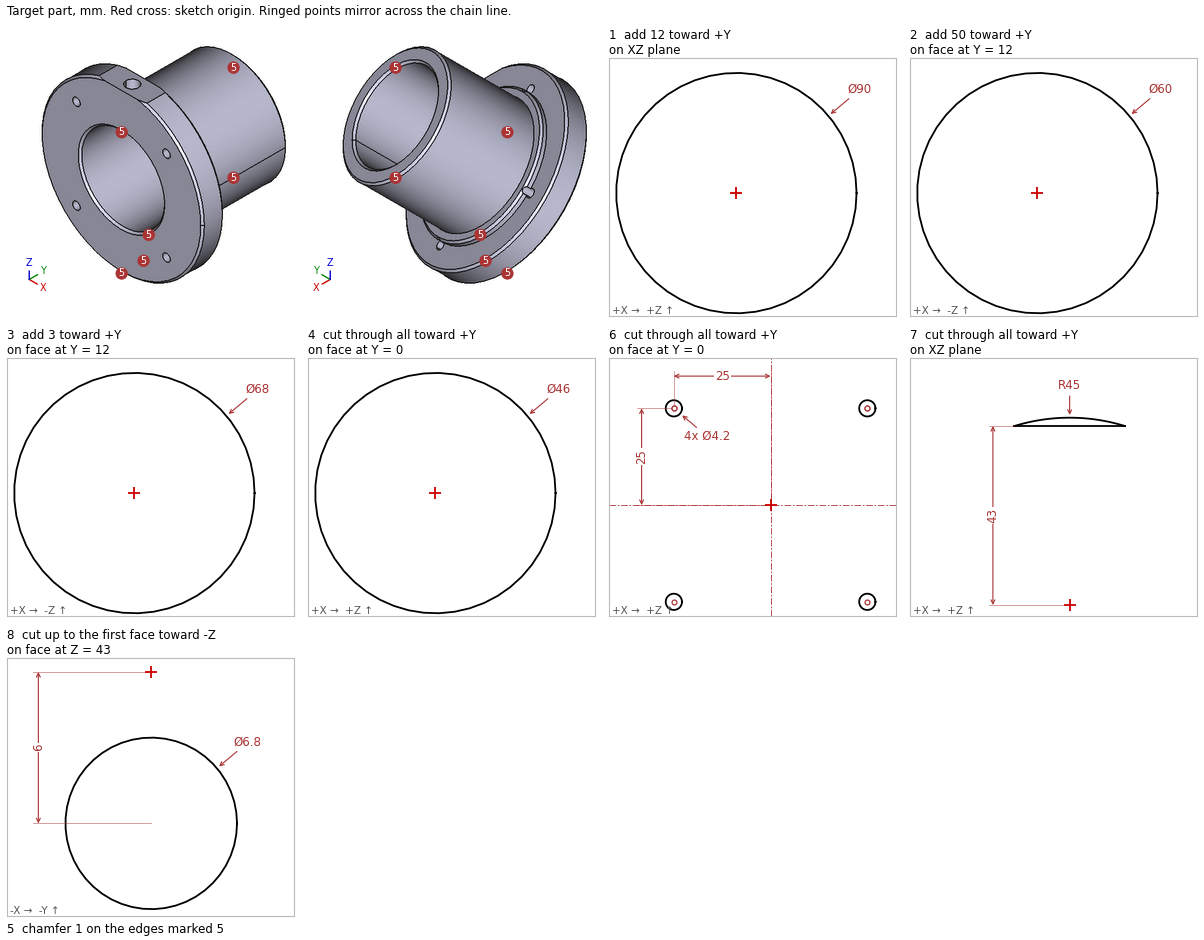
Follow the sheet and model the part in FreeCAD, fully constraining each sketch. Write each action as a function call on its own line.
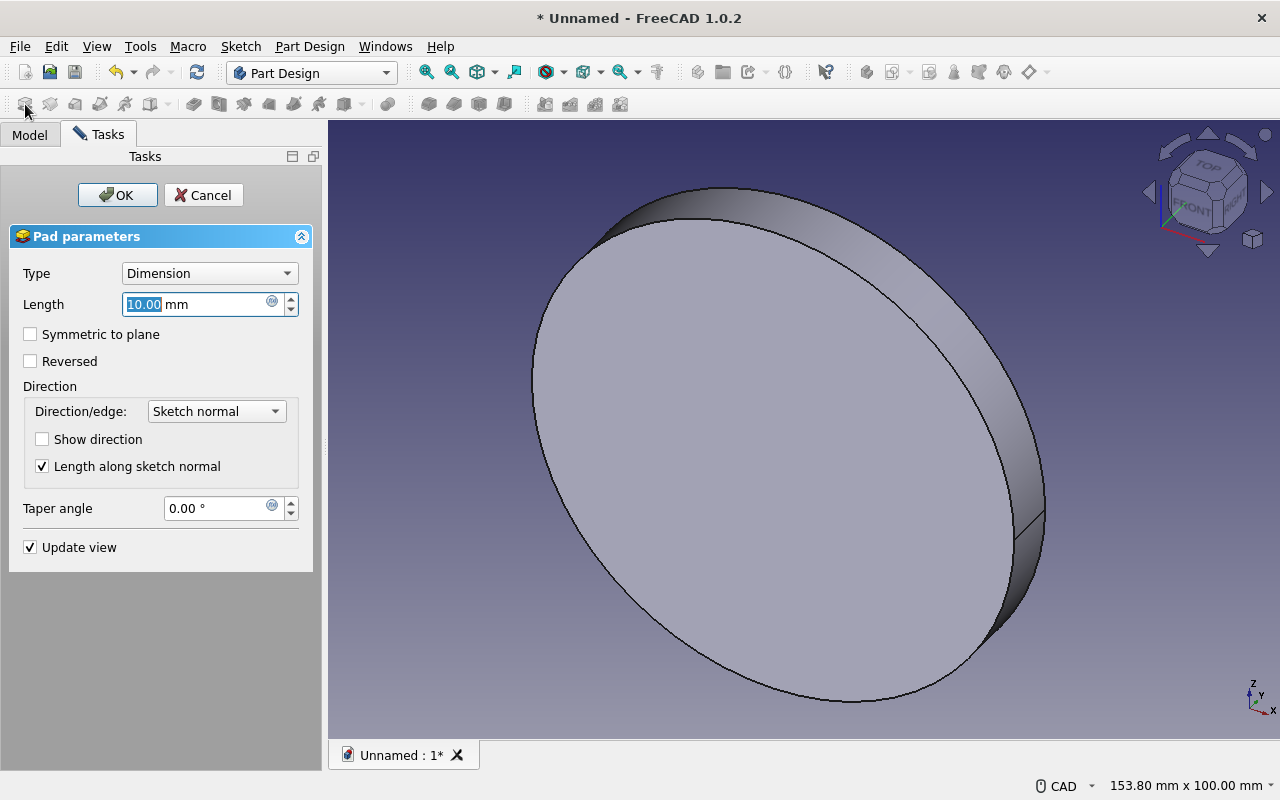
text(12)
key(Tab)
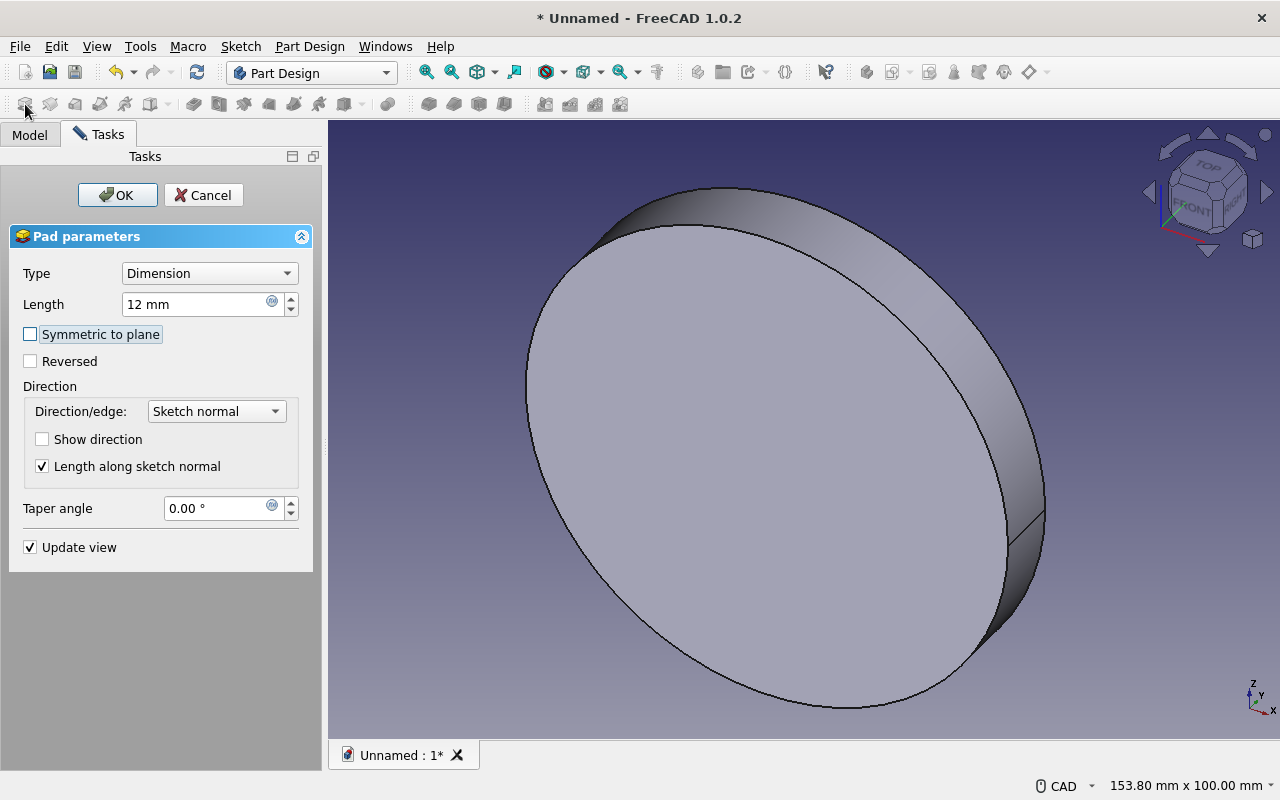
click(31, 361)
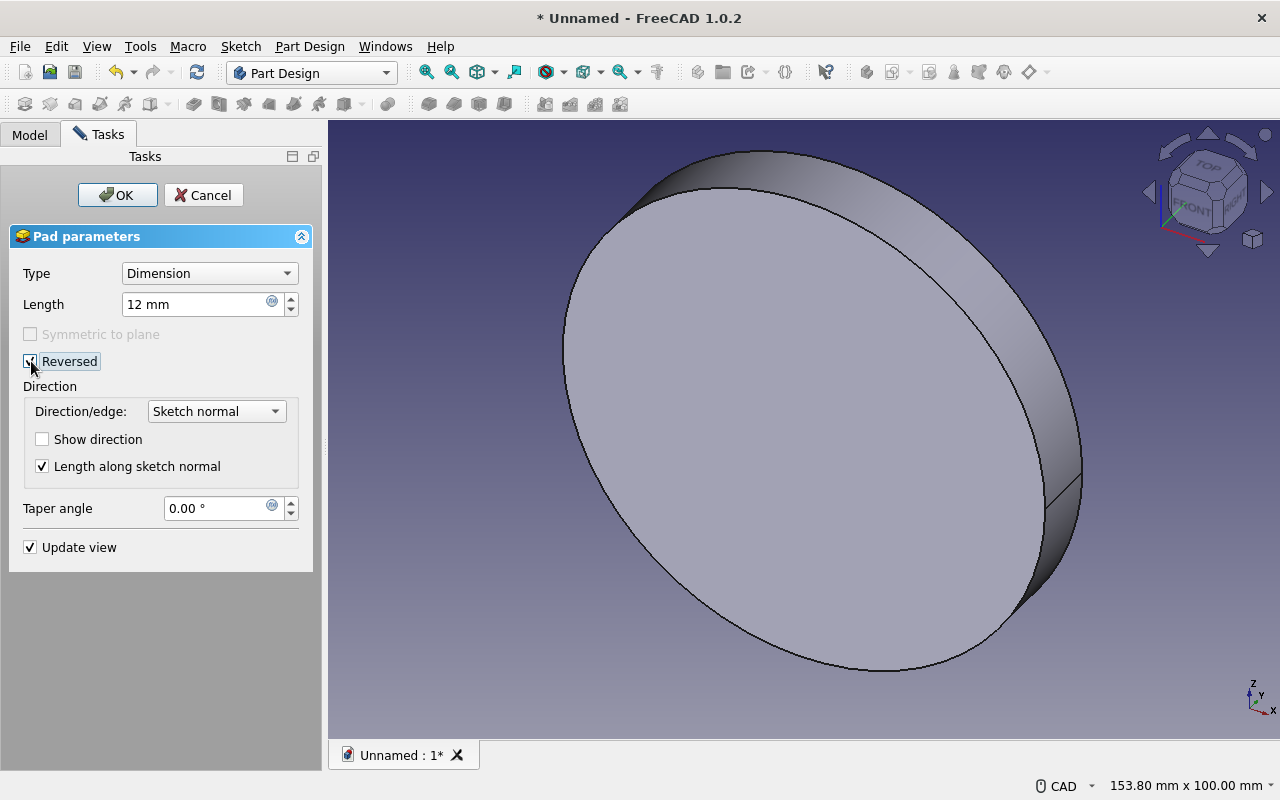
click(118, 195)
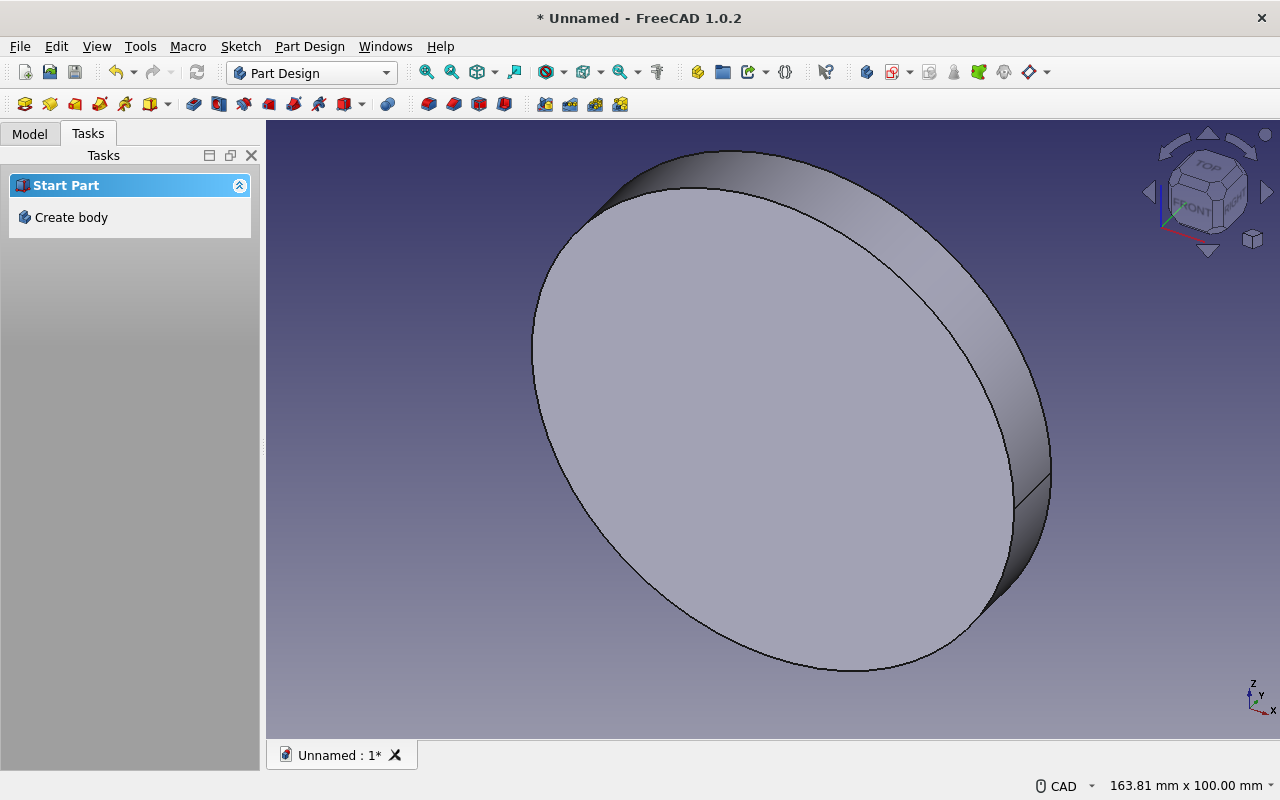
click(427, 72)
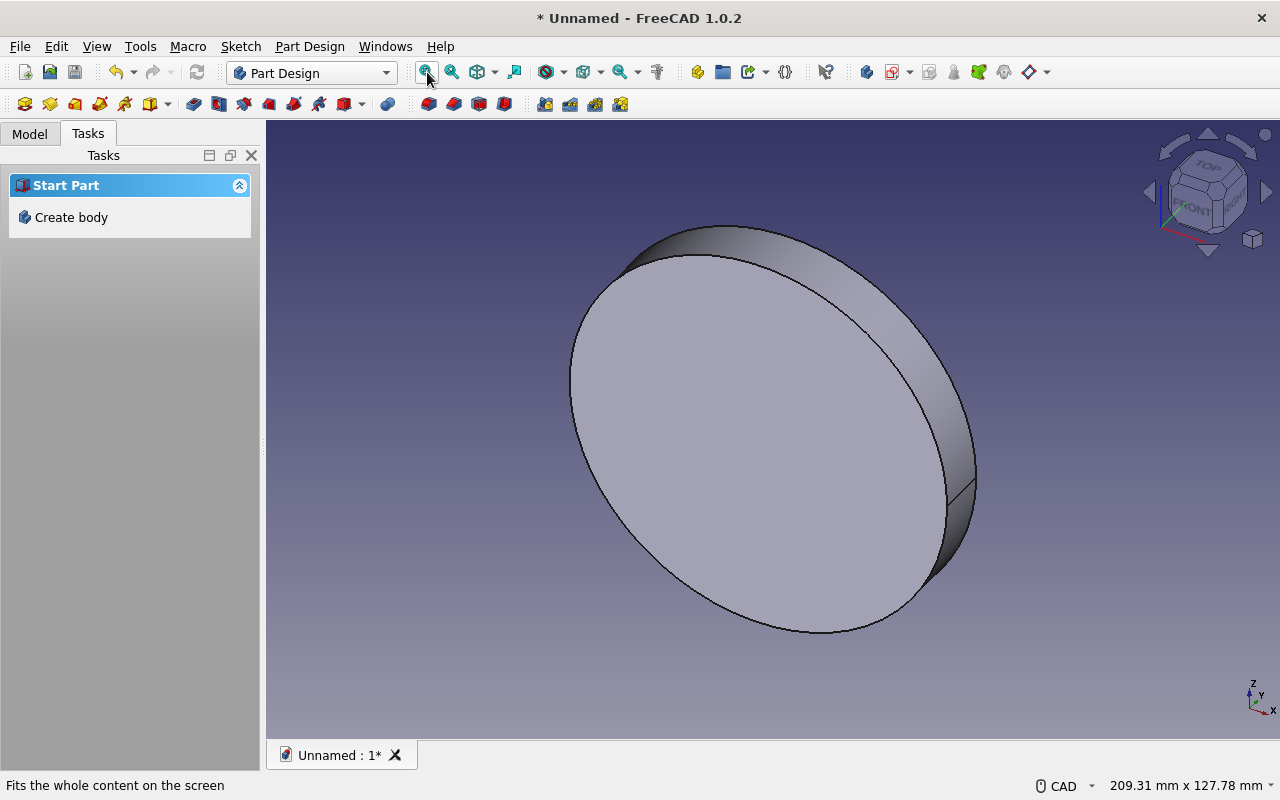
key(4)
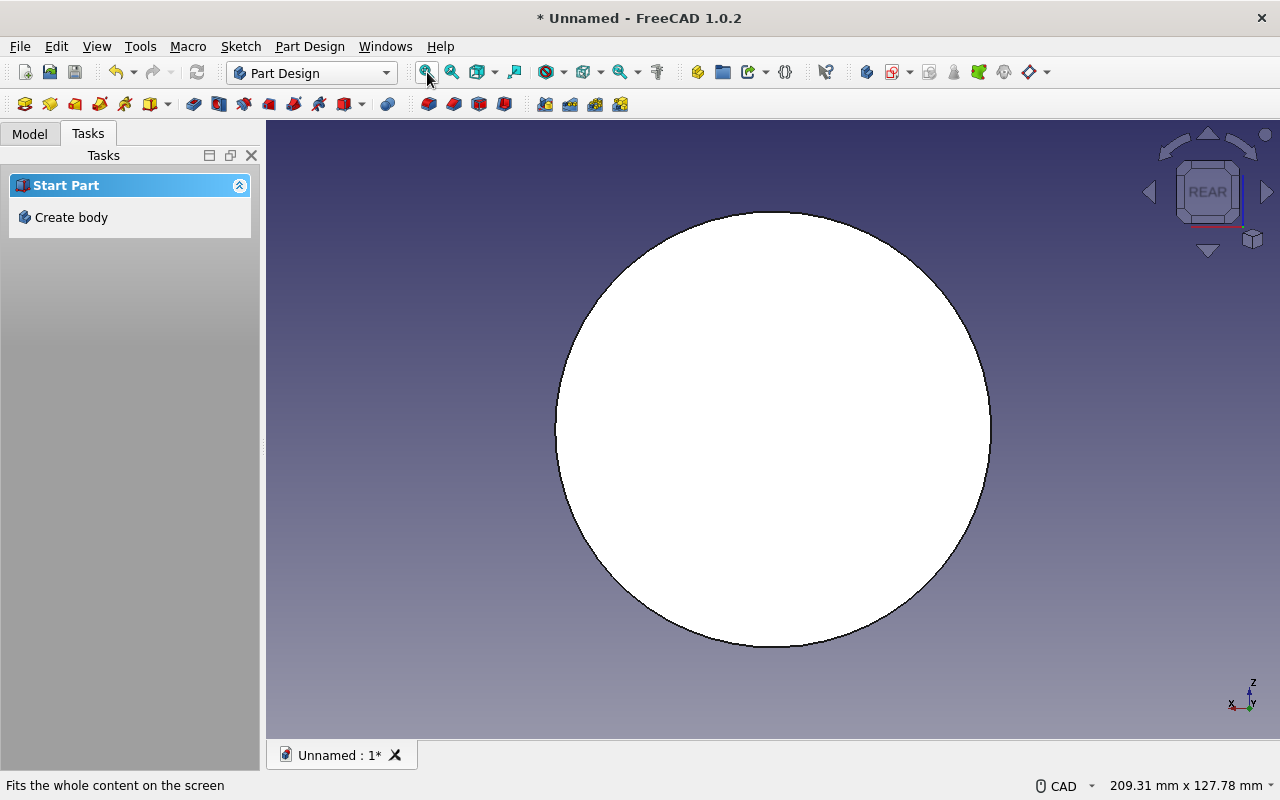
click(773, 428)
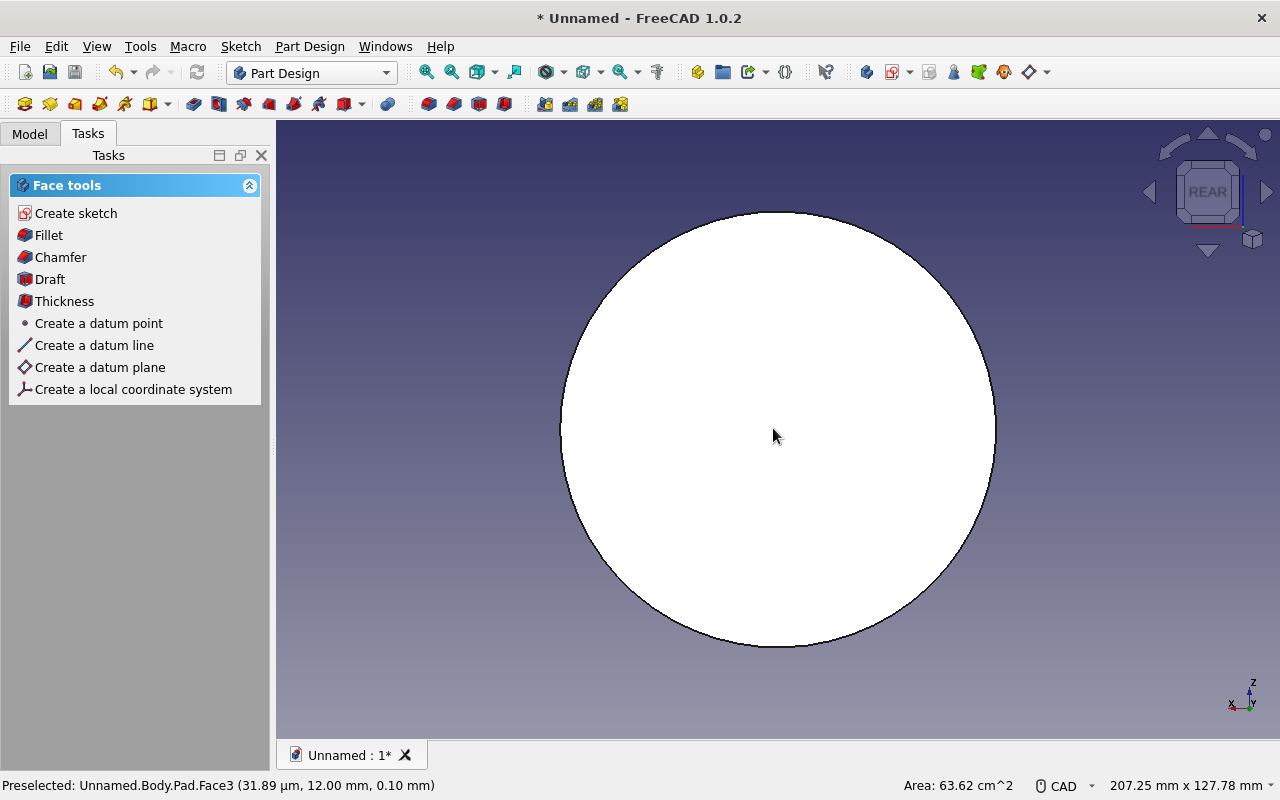
click(892, 72)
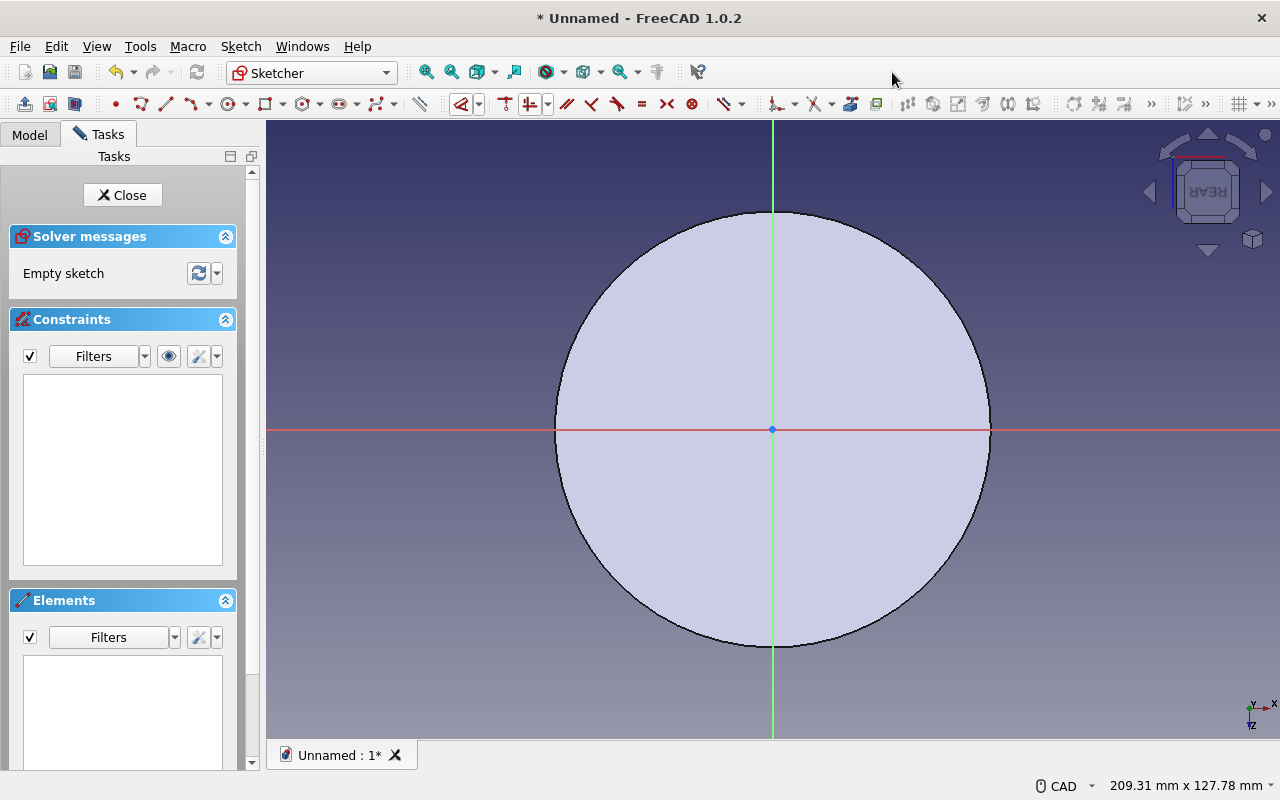
scroll(912, 430, up, 2)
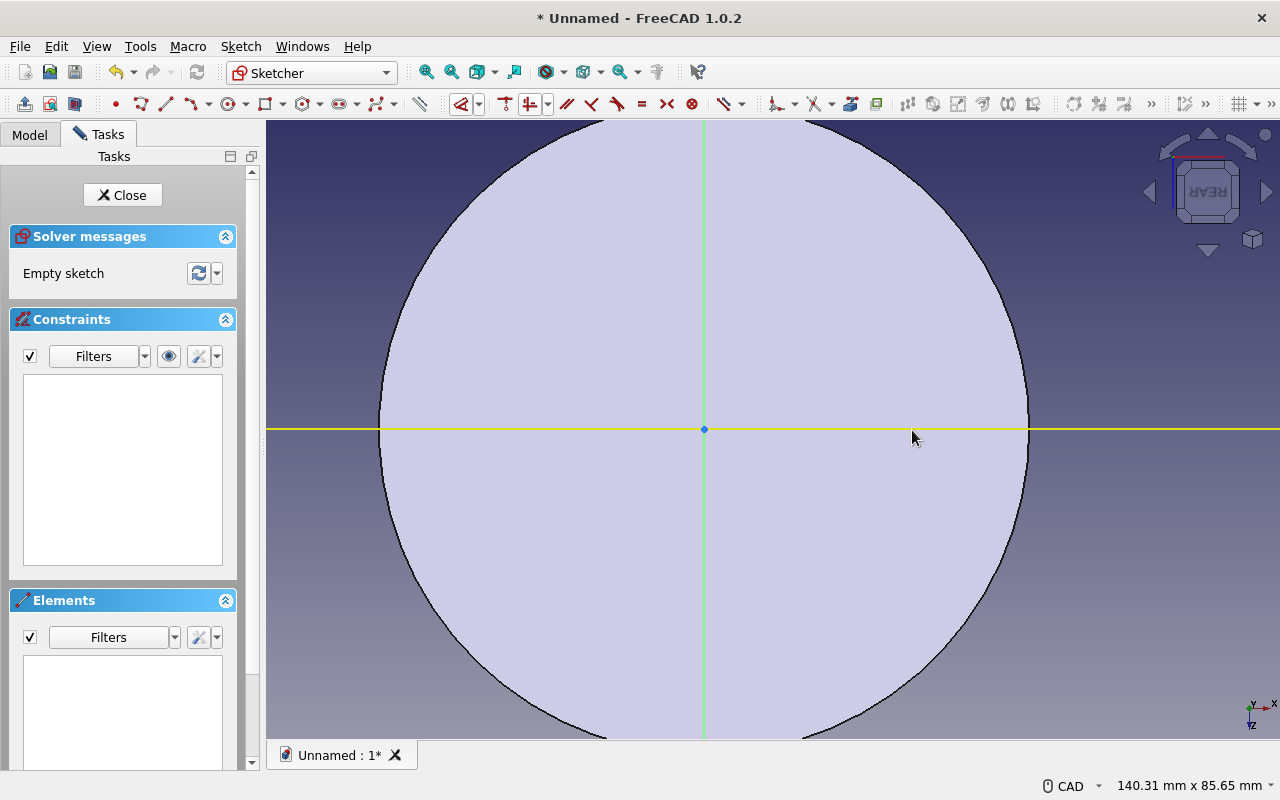
click(228, 104)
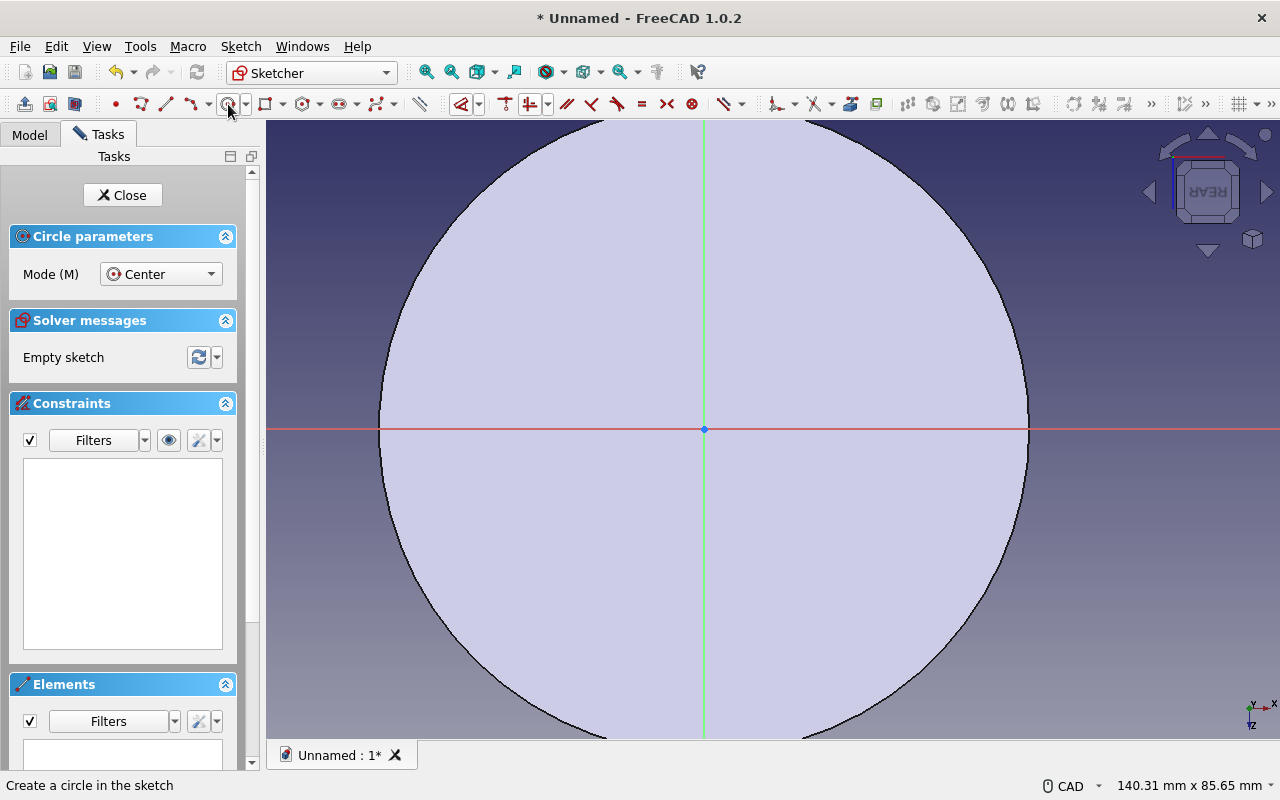
click(704, 429)
move(857, 276)